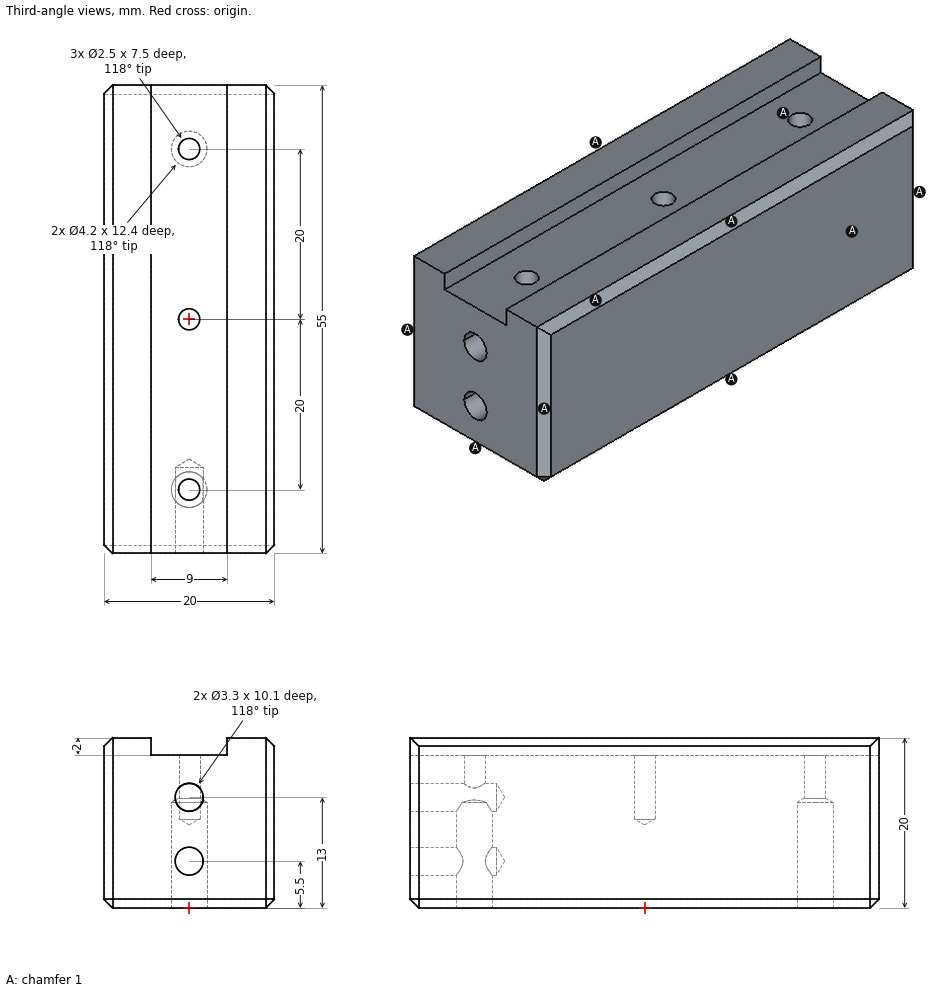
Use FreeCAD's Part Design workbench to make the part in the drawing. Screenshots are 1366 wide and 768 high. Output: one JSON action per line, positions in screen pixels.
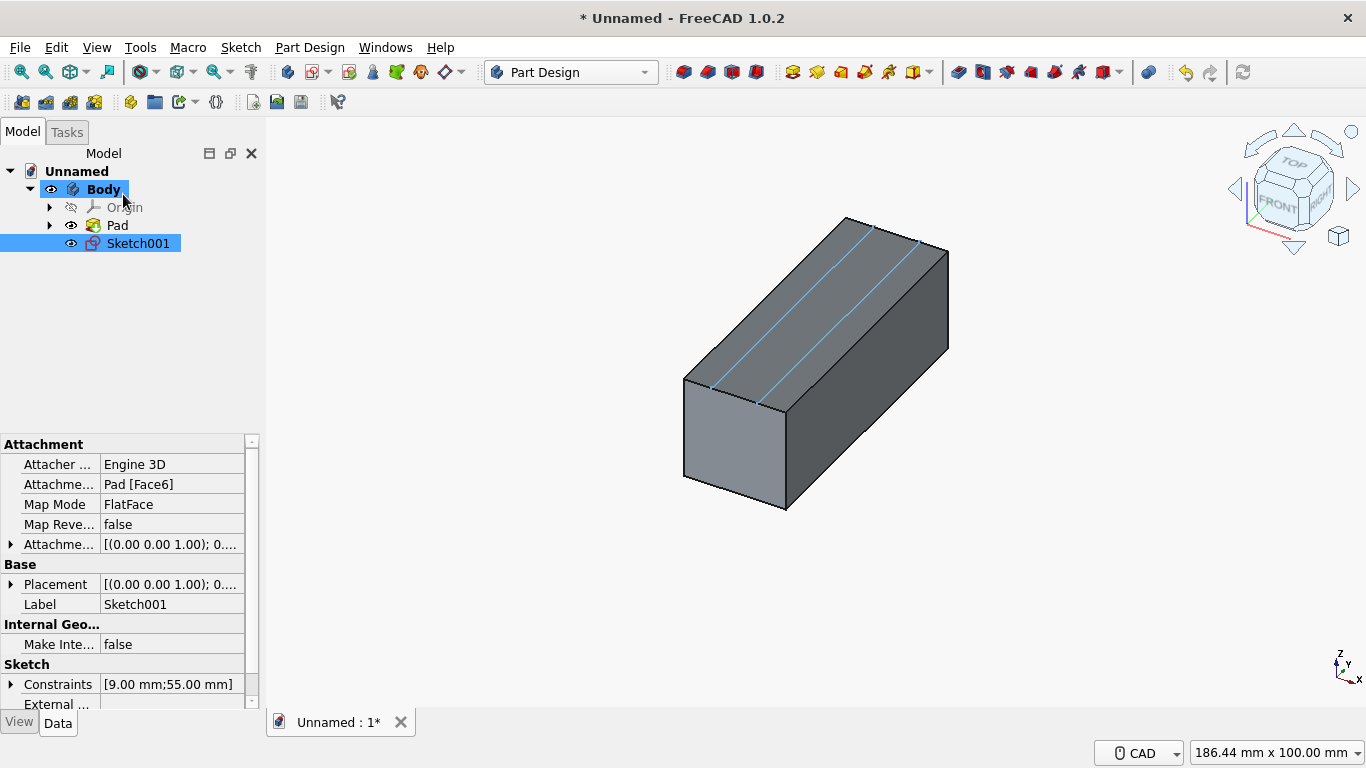
{"action": "left_click", "coordinate": [960, 72]}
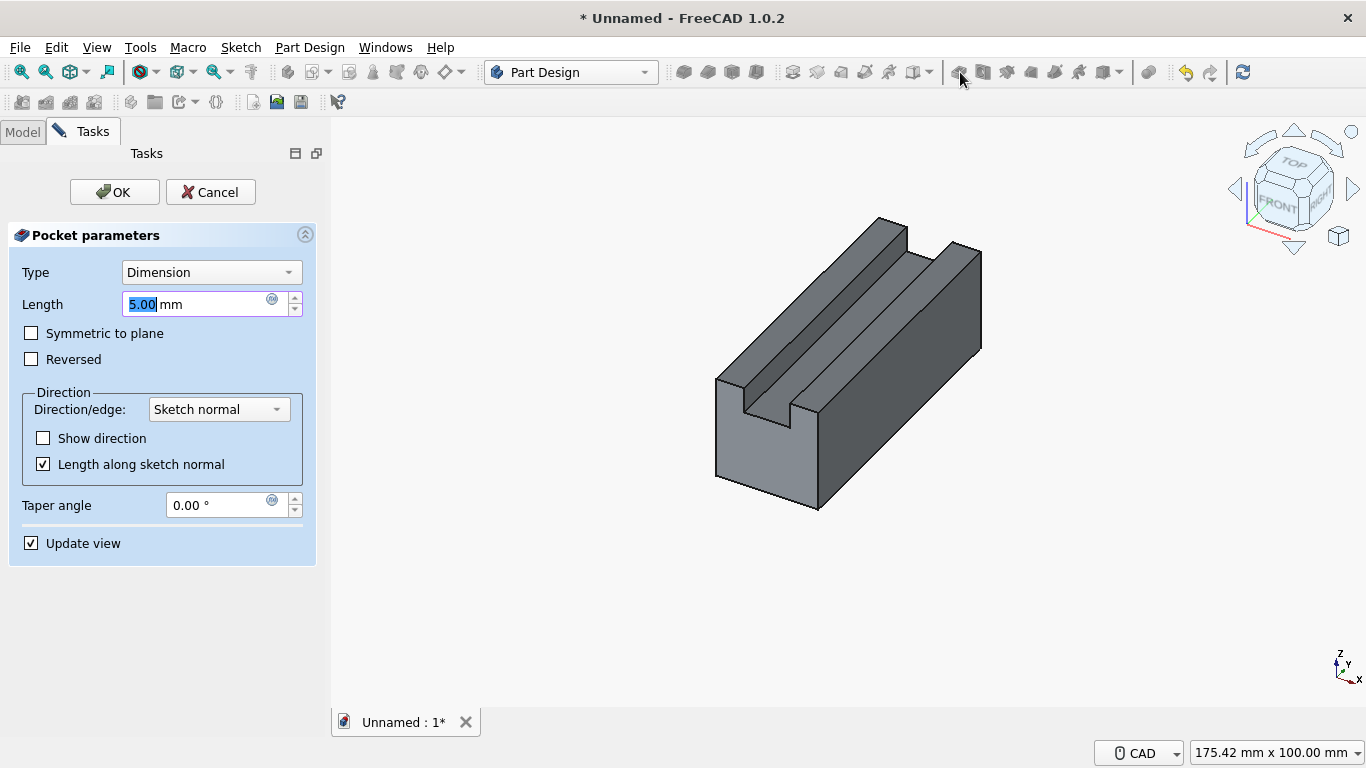
{"action": "type", "text": "2"}
{"action": "key", "text": "Tab"}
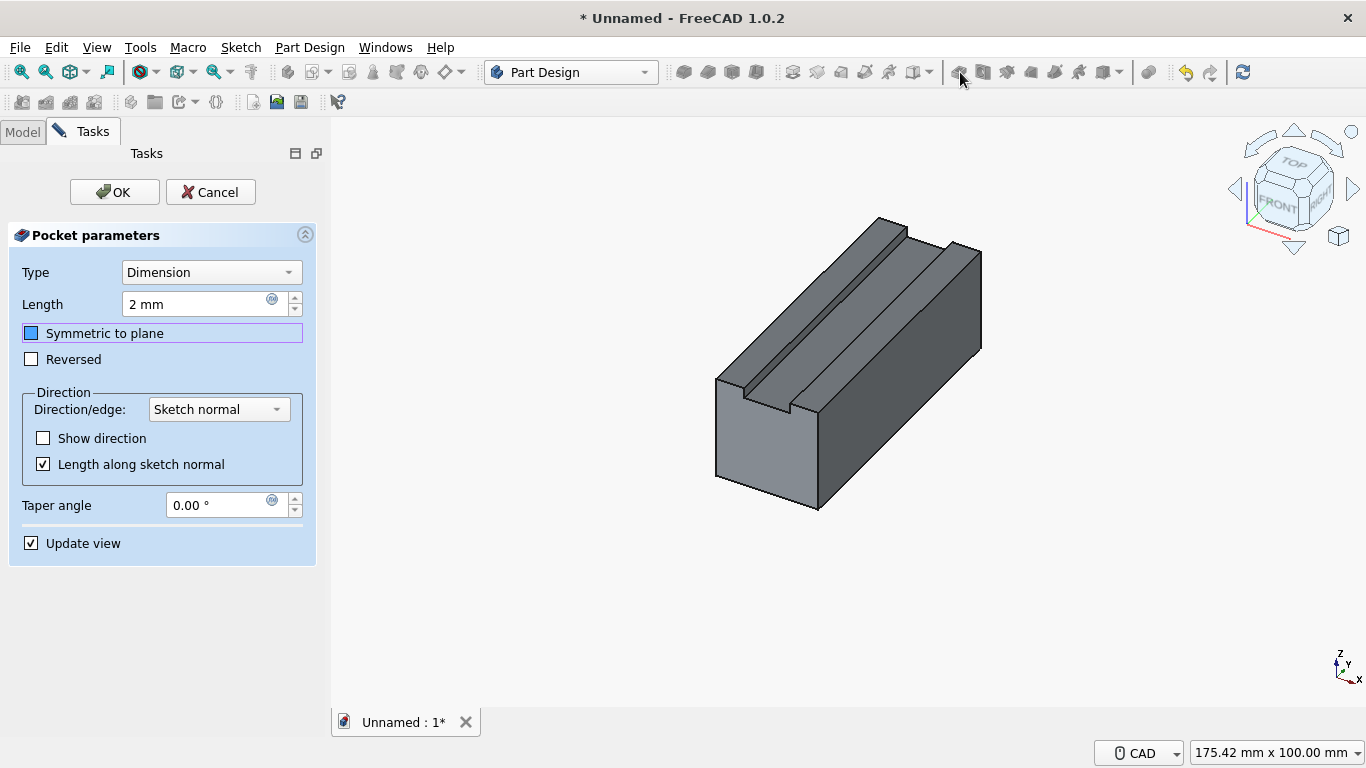
{"action": "left_click", "coordinate": [115, 192]}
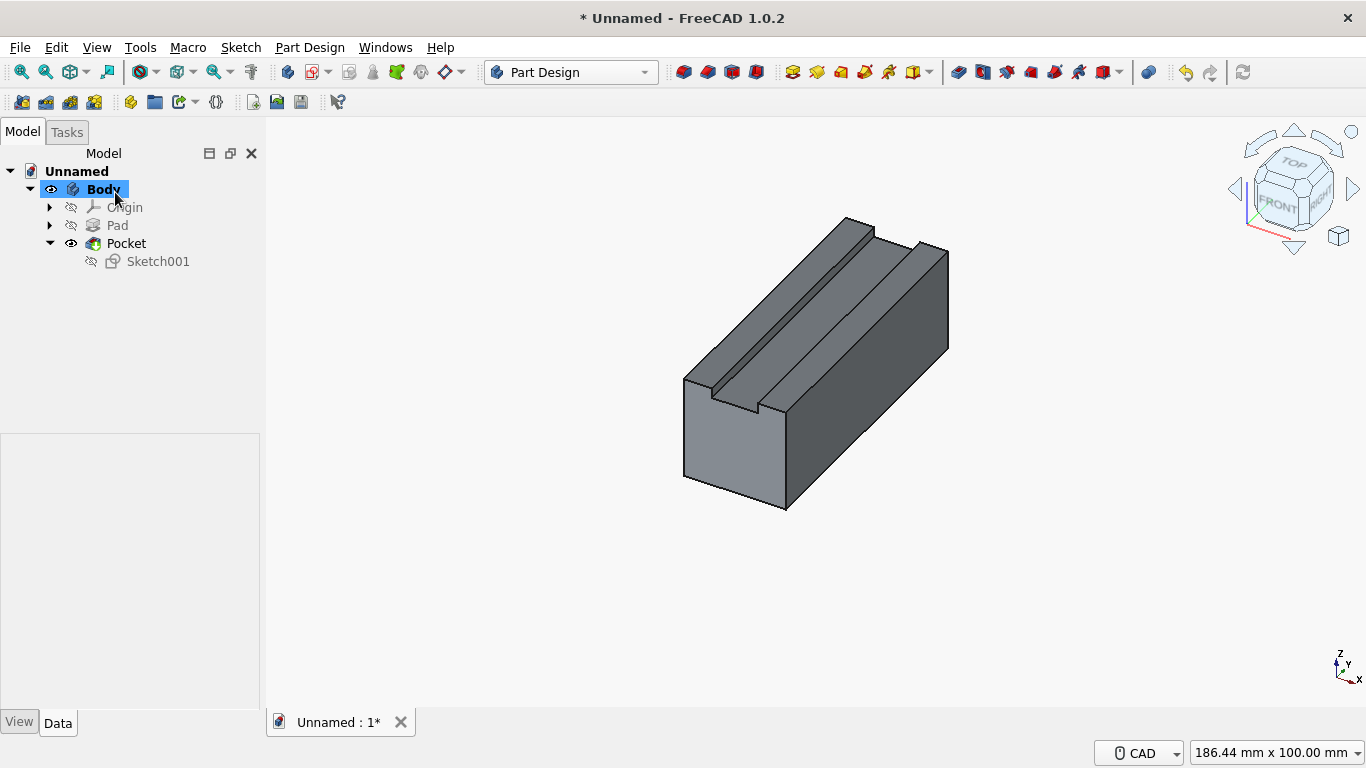
{"action": "left_click", "coordinate": [862, 278]}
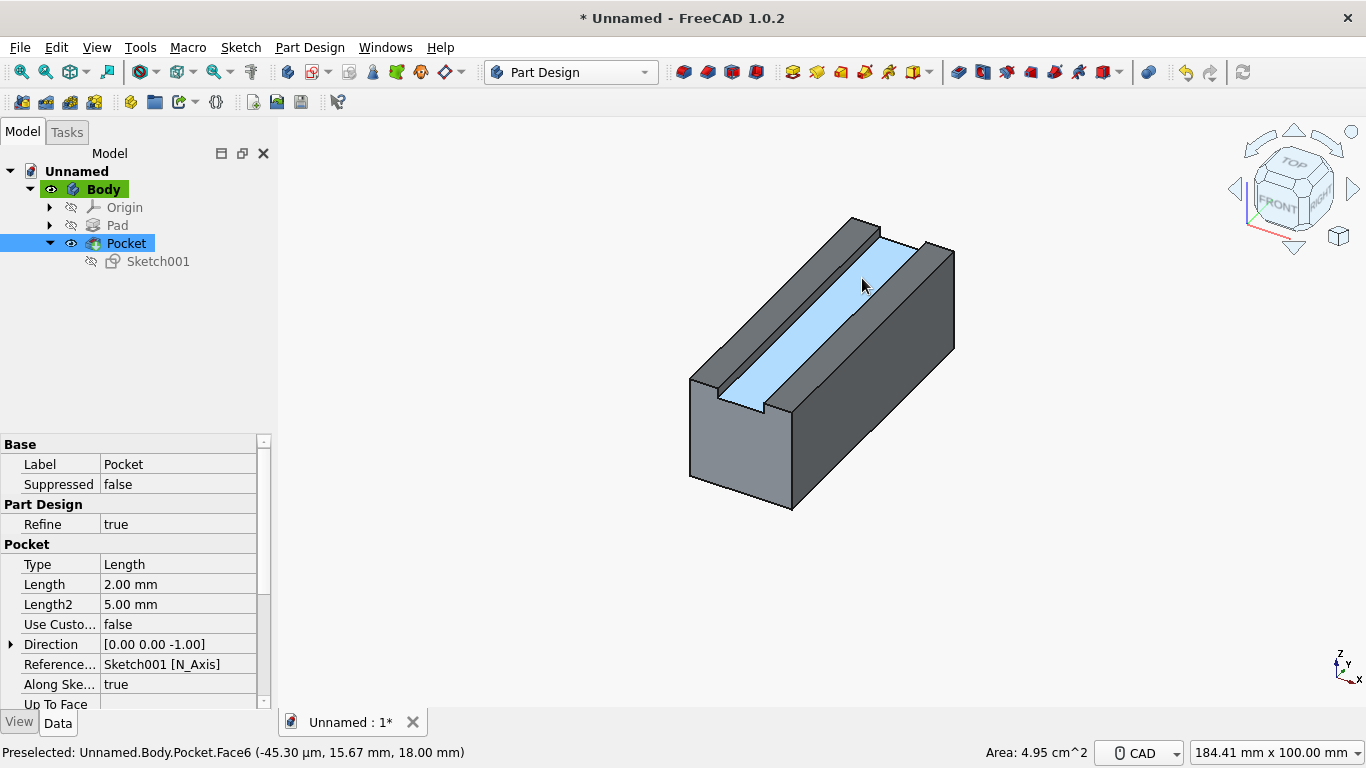
{"action": "left_click", "coordinate": [312, 72]}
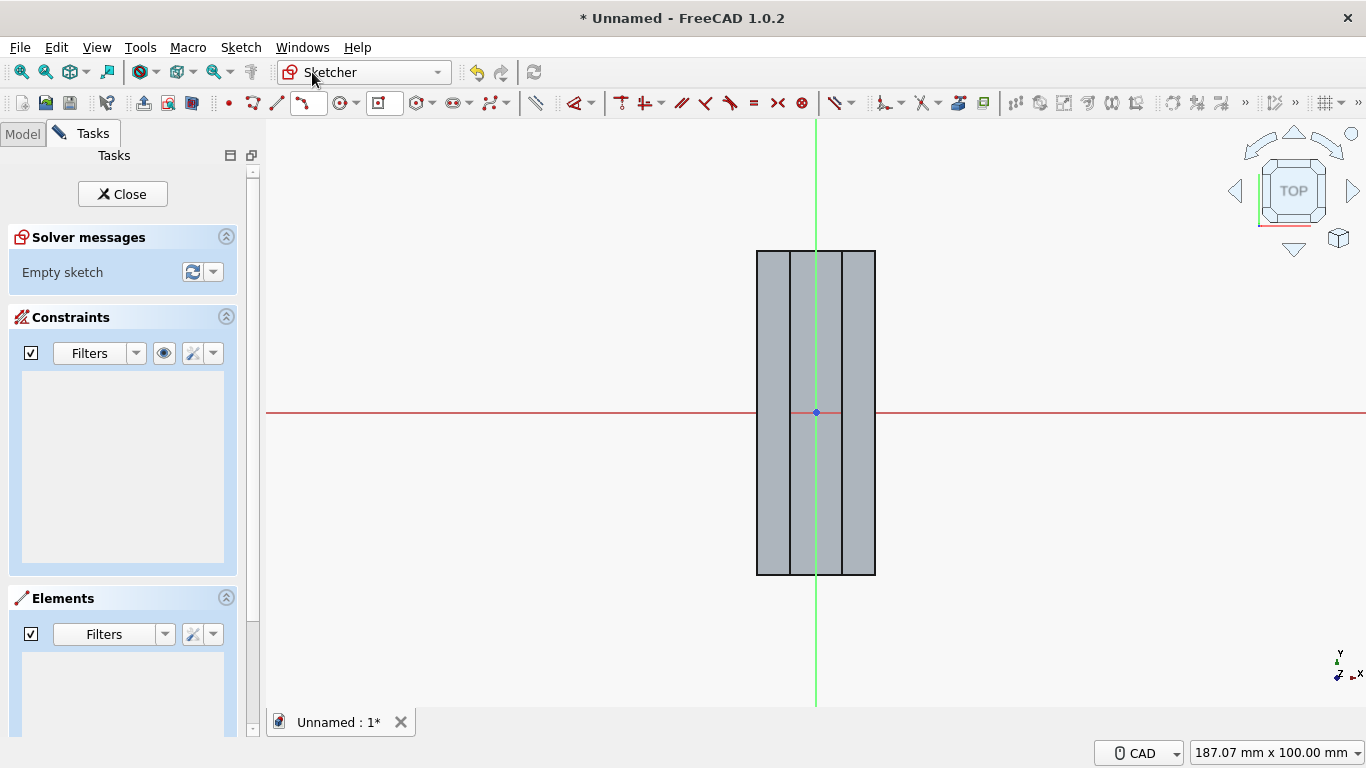
{"action": "scroll", "coordinate": [955, 413], "scroll_direction": "up", "scroll_amount": 2}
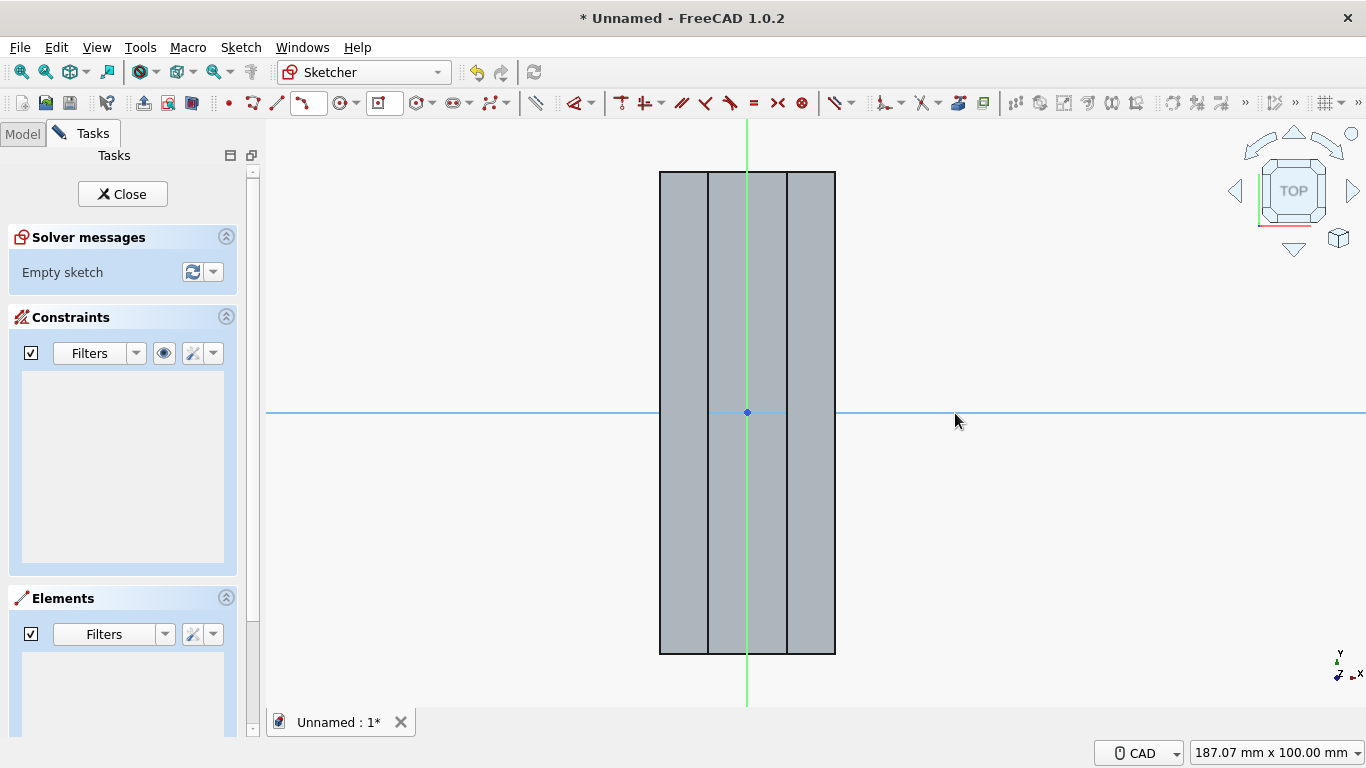
{"action": "left_click", "coordinate": [340, 104]}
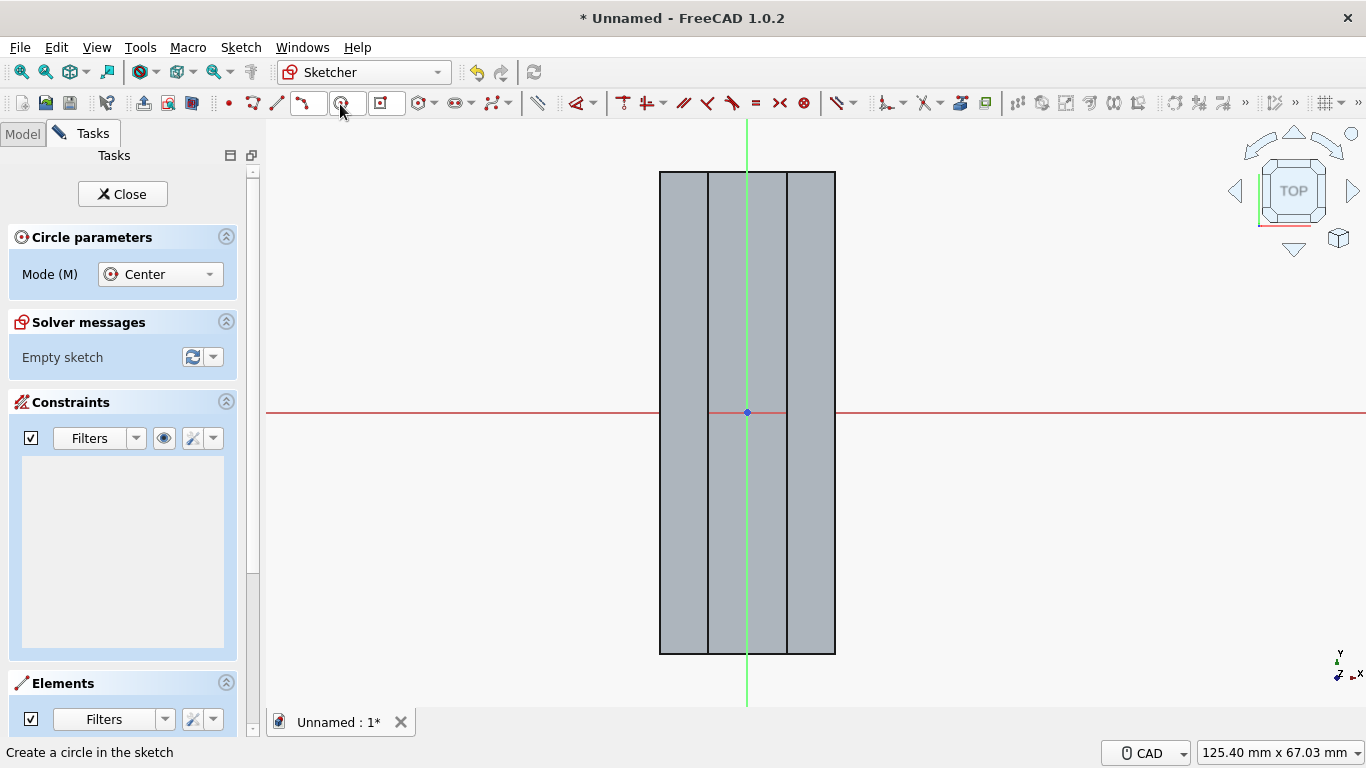
{"action": "scroll", "coordinate": [747, 237], "scroll_direction": "up", "scroll_amount": 4}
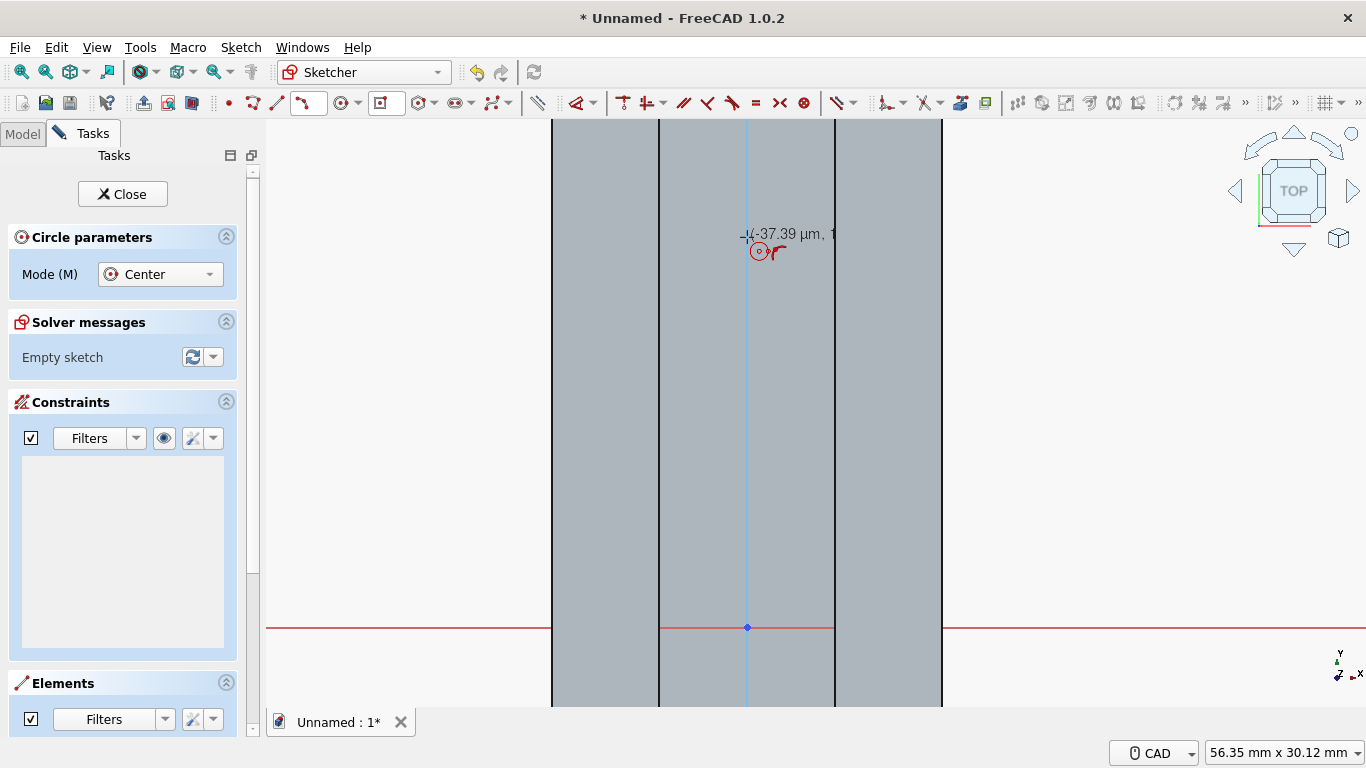
{"action": "left_click", "coordinate": [747, 237]}
{"action": "mouse_move", "coordinate": [764, 220]}